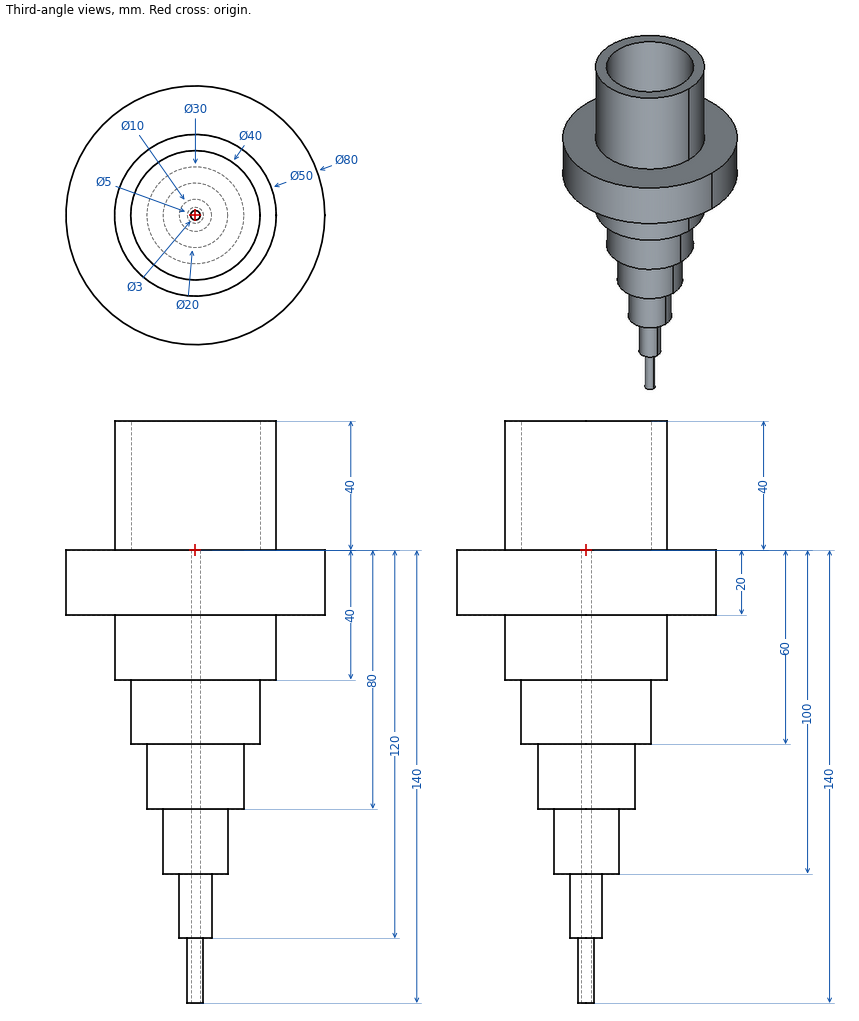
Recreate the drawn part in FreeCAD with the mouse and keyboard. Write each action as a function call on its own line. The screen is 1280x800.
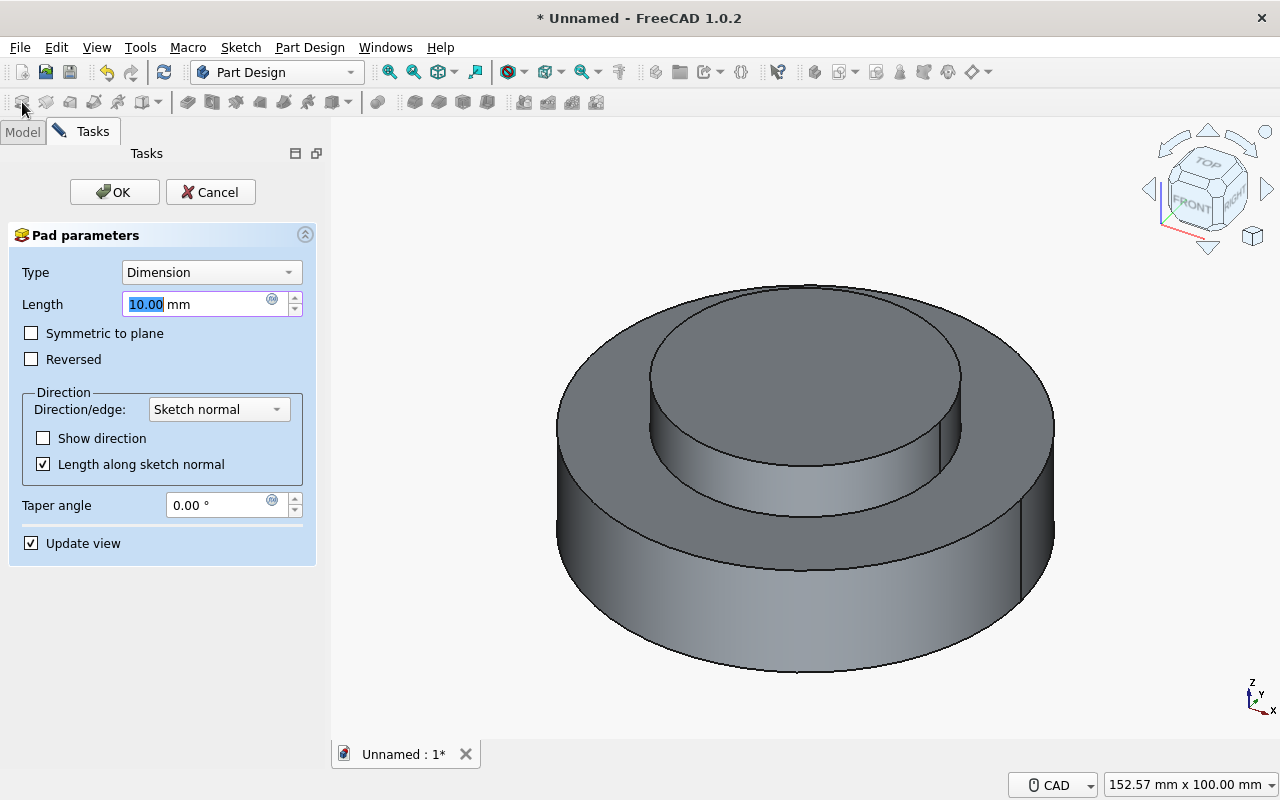
text(40)
key(Tab)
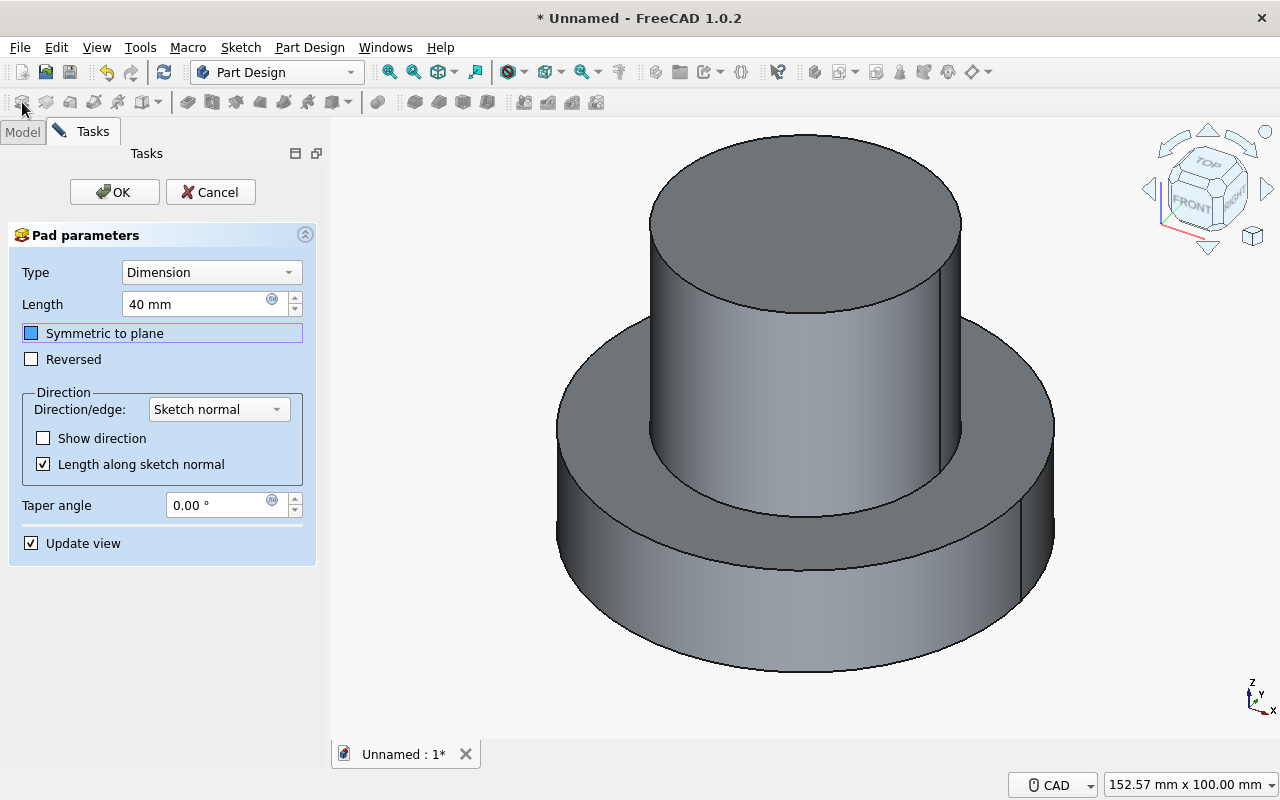
click(30, 359)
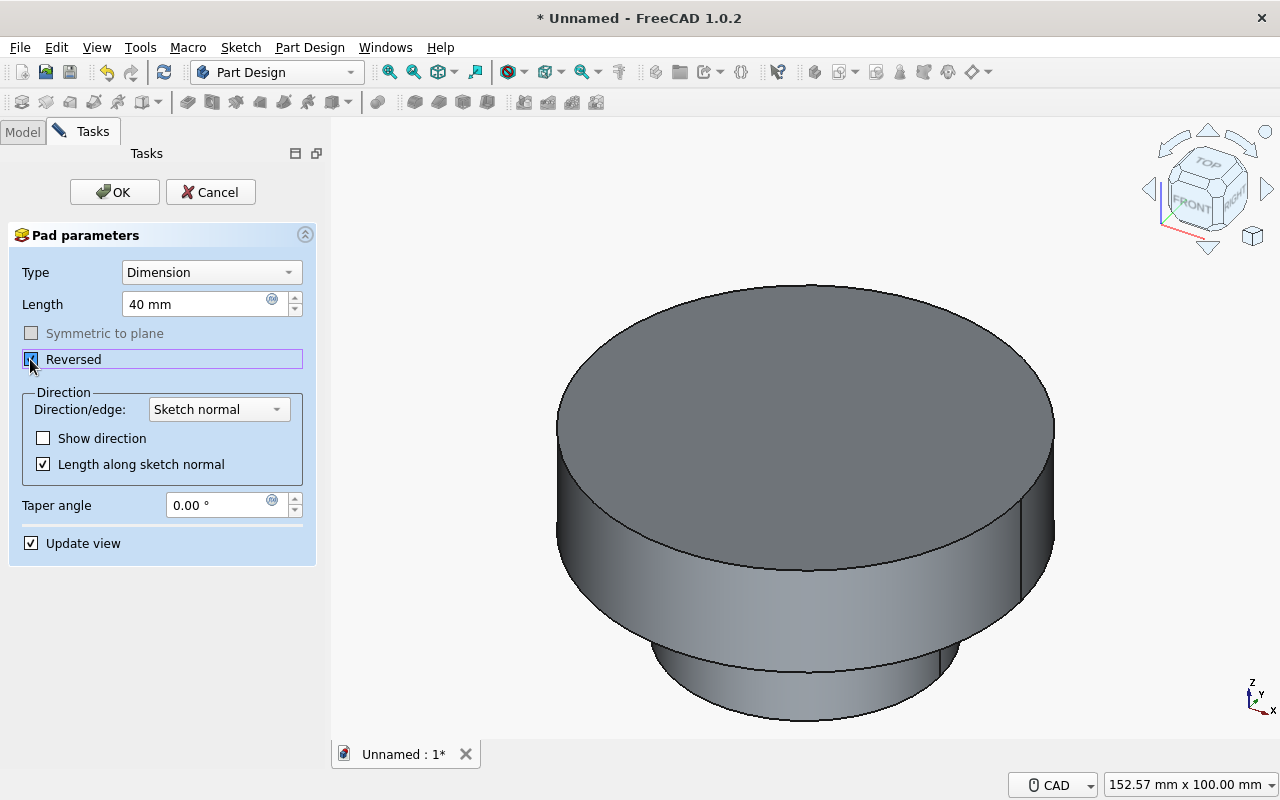
click(115, 192)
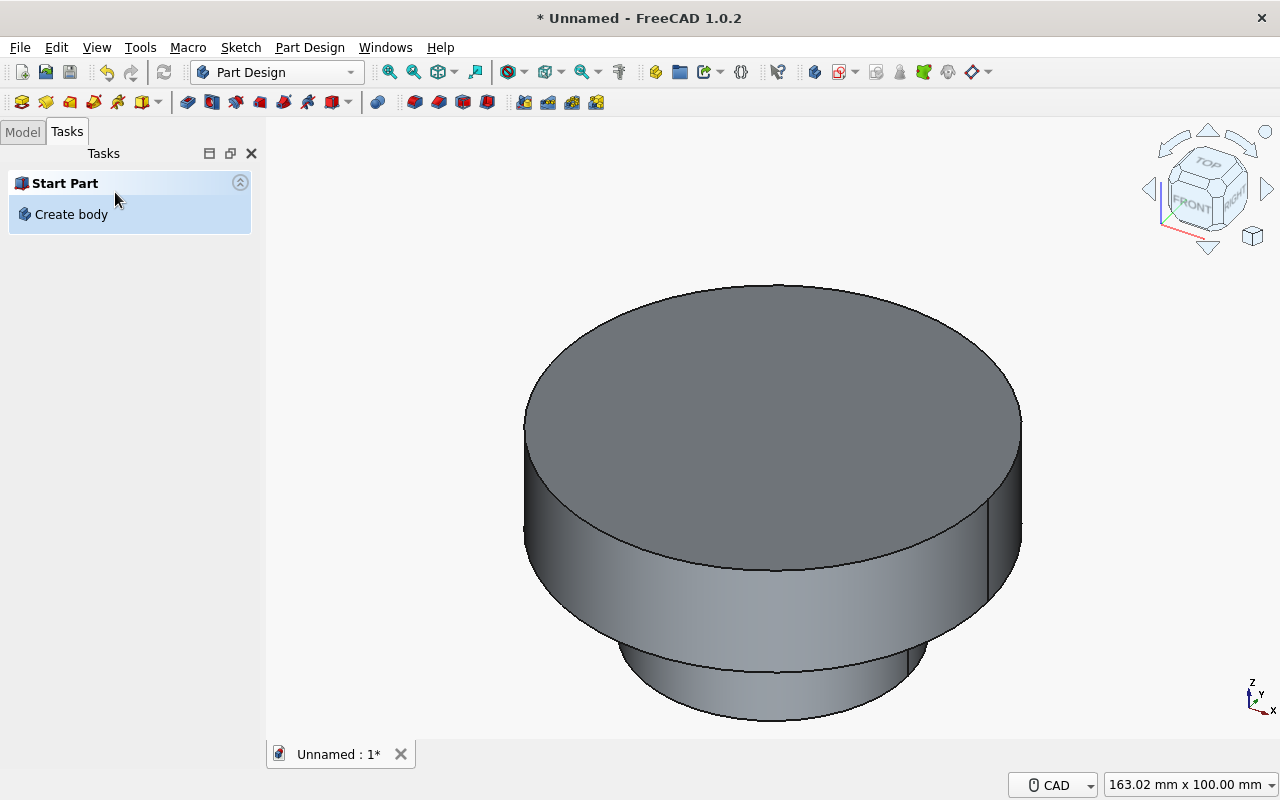
key(v)
key(f)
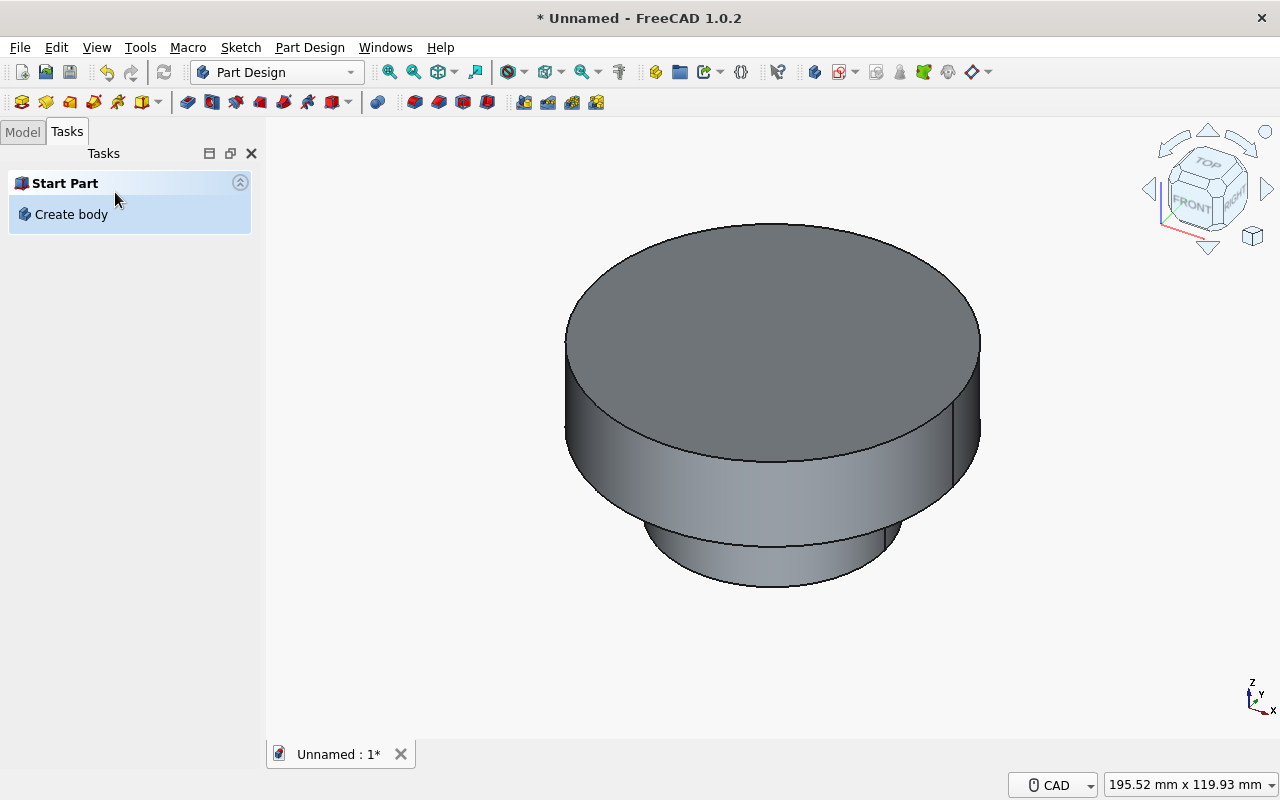
click(773, 342)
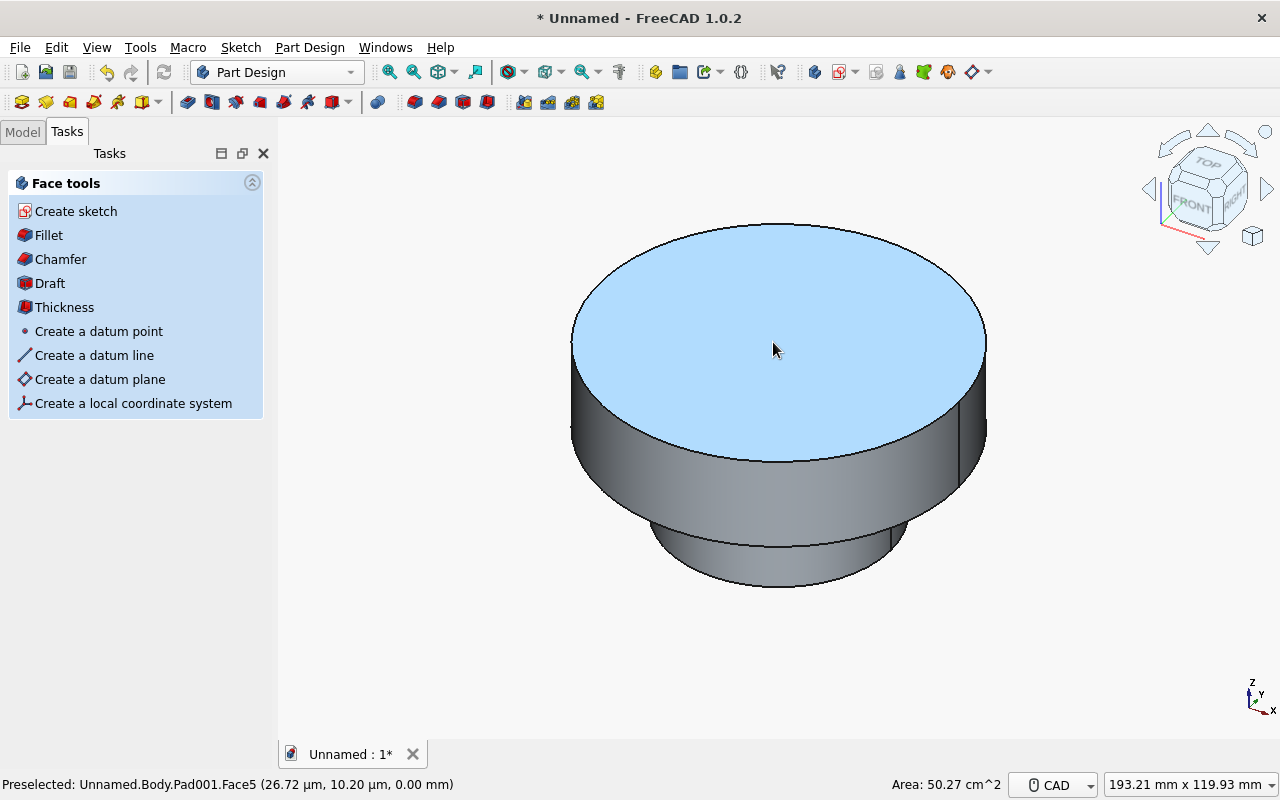
click(840, 72)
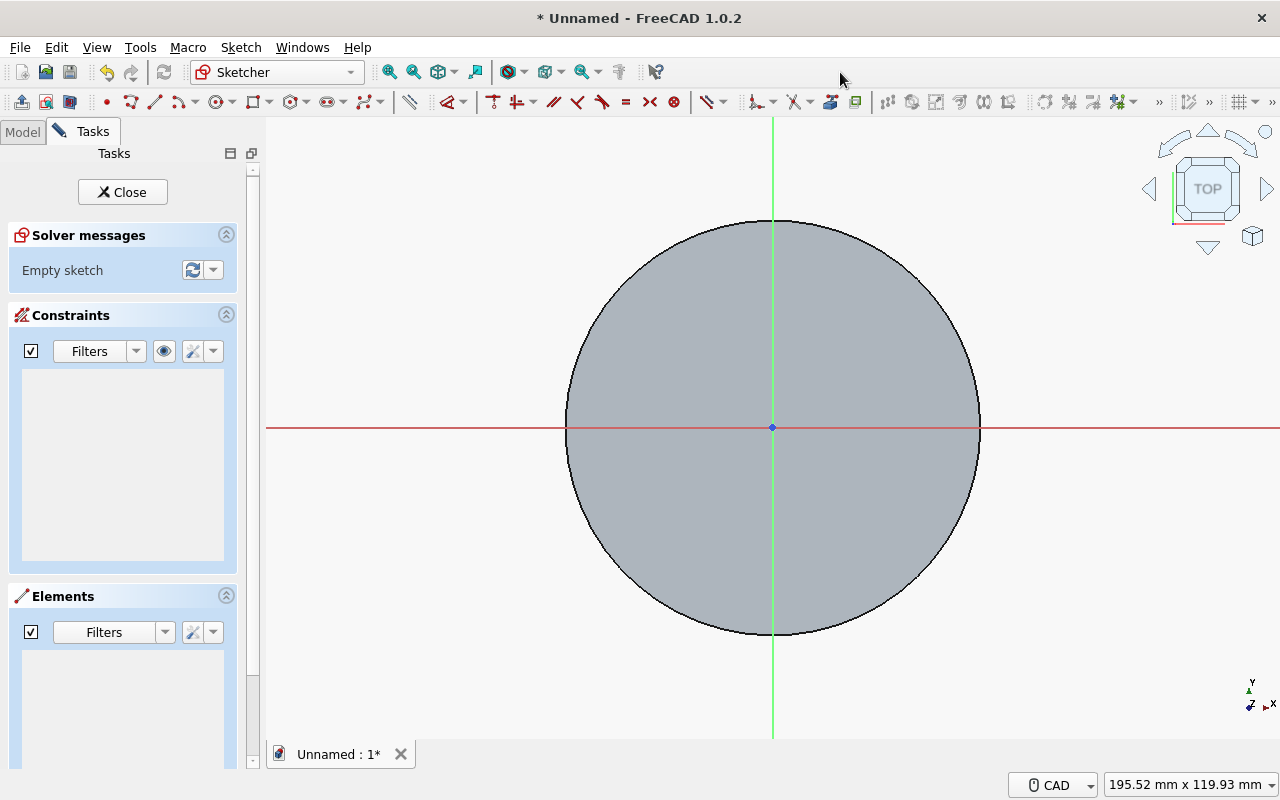
scroll(856, 428, up, 3)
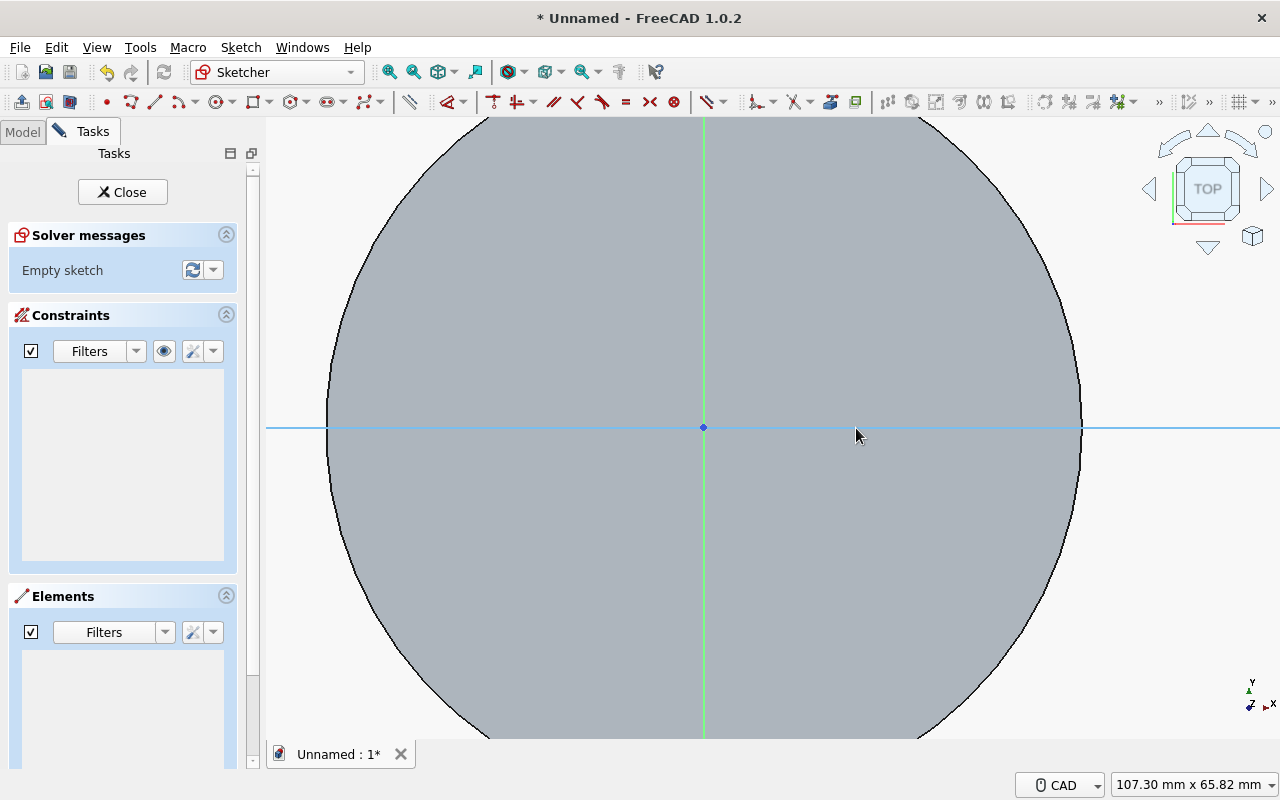
click(216, 102)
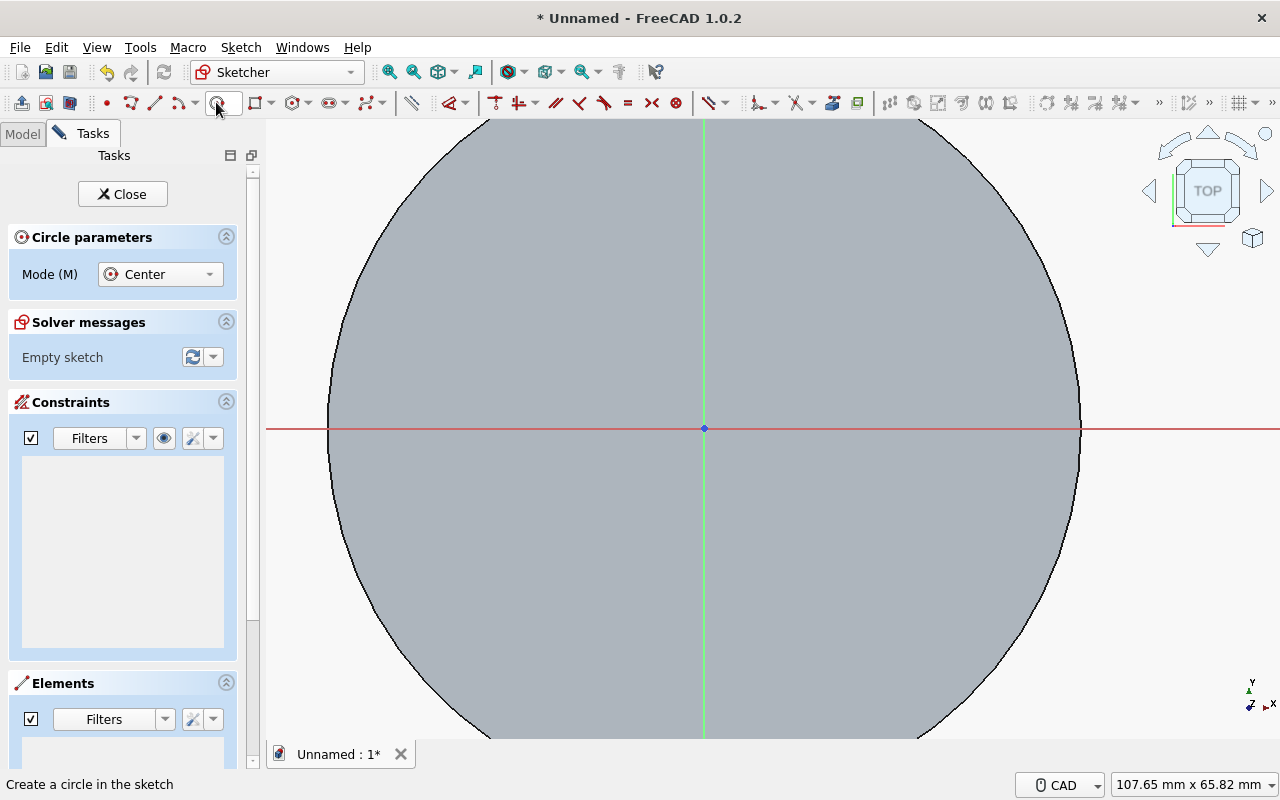
click(704, 429)
move(837, 295)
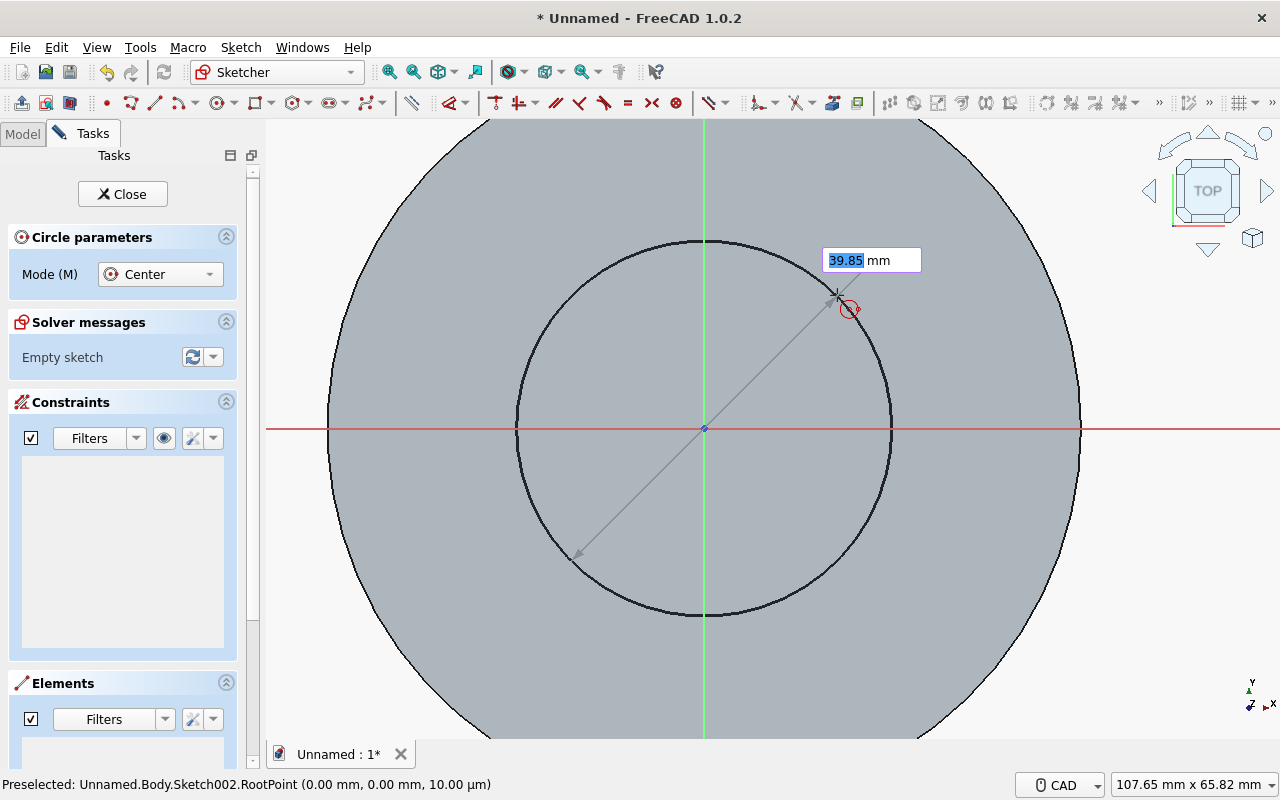
text(40)
key(Return)
key(Escape)